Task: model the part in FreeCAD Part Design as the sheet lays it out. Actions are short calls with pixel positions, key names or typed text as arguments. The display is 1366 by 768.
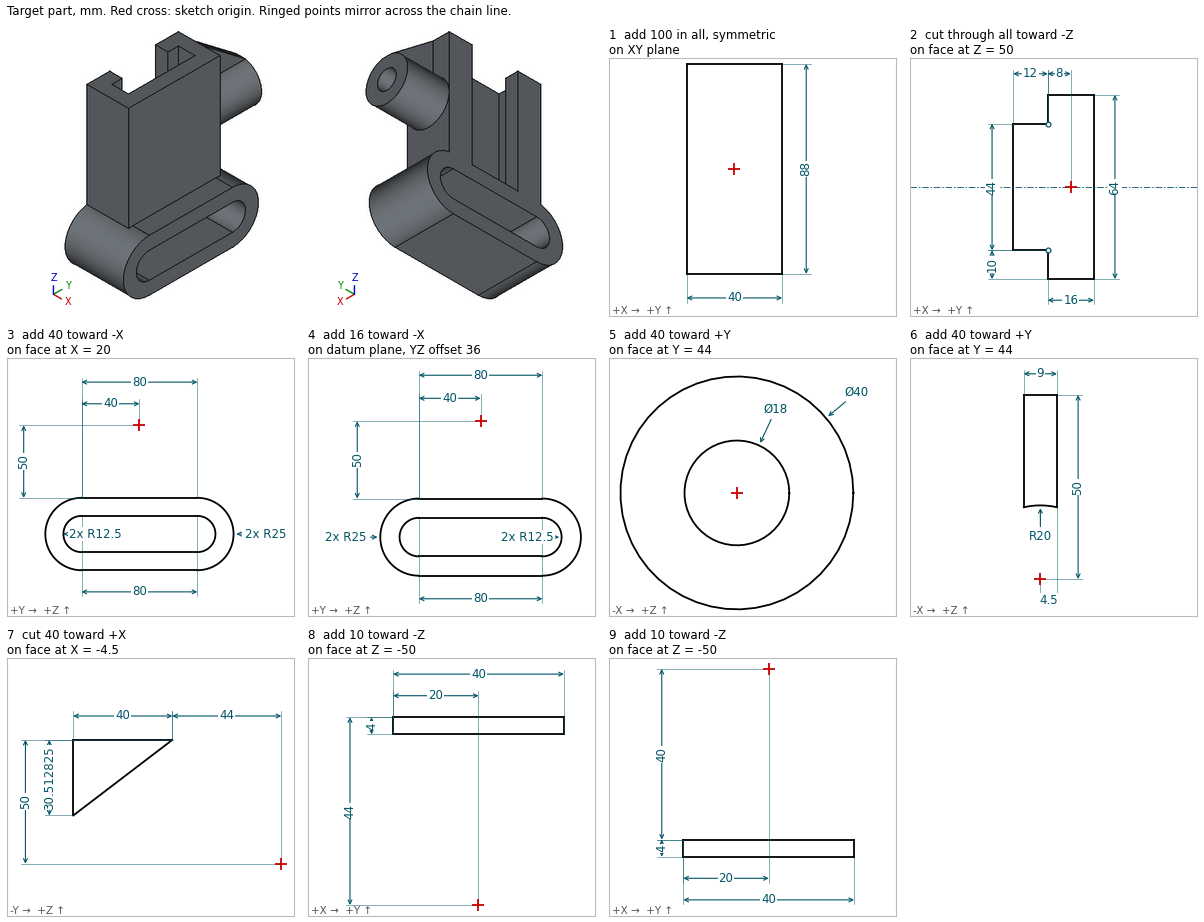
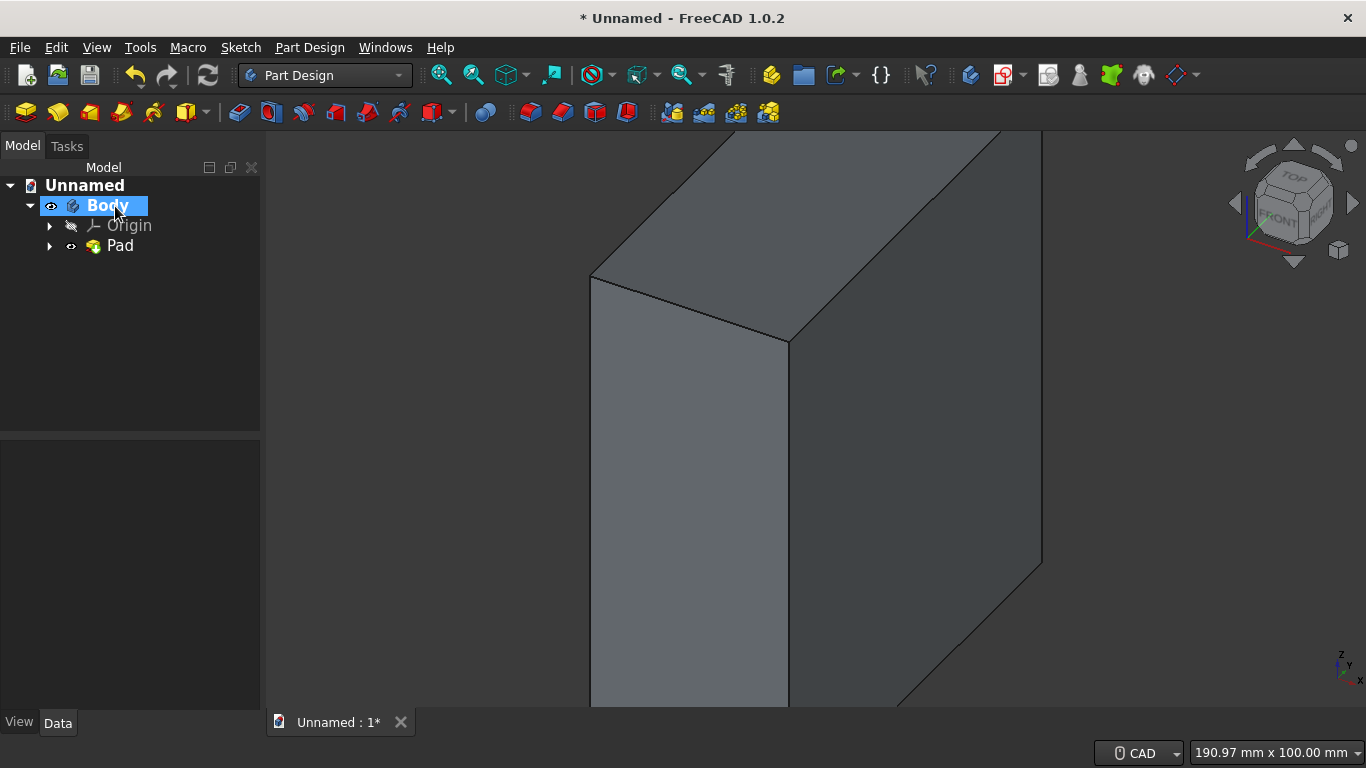
click(442, 76)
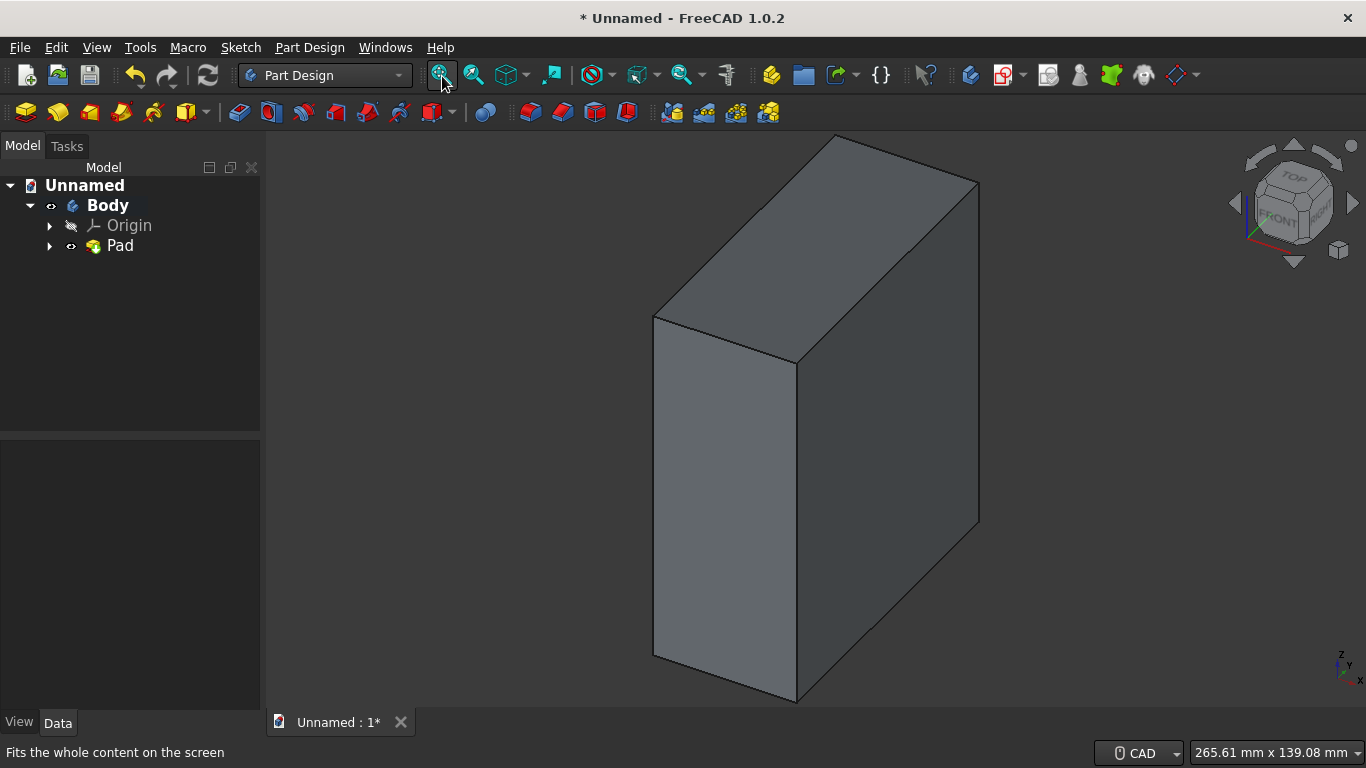
click(842, 223)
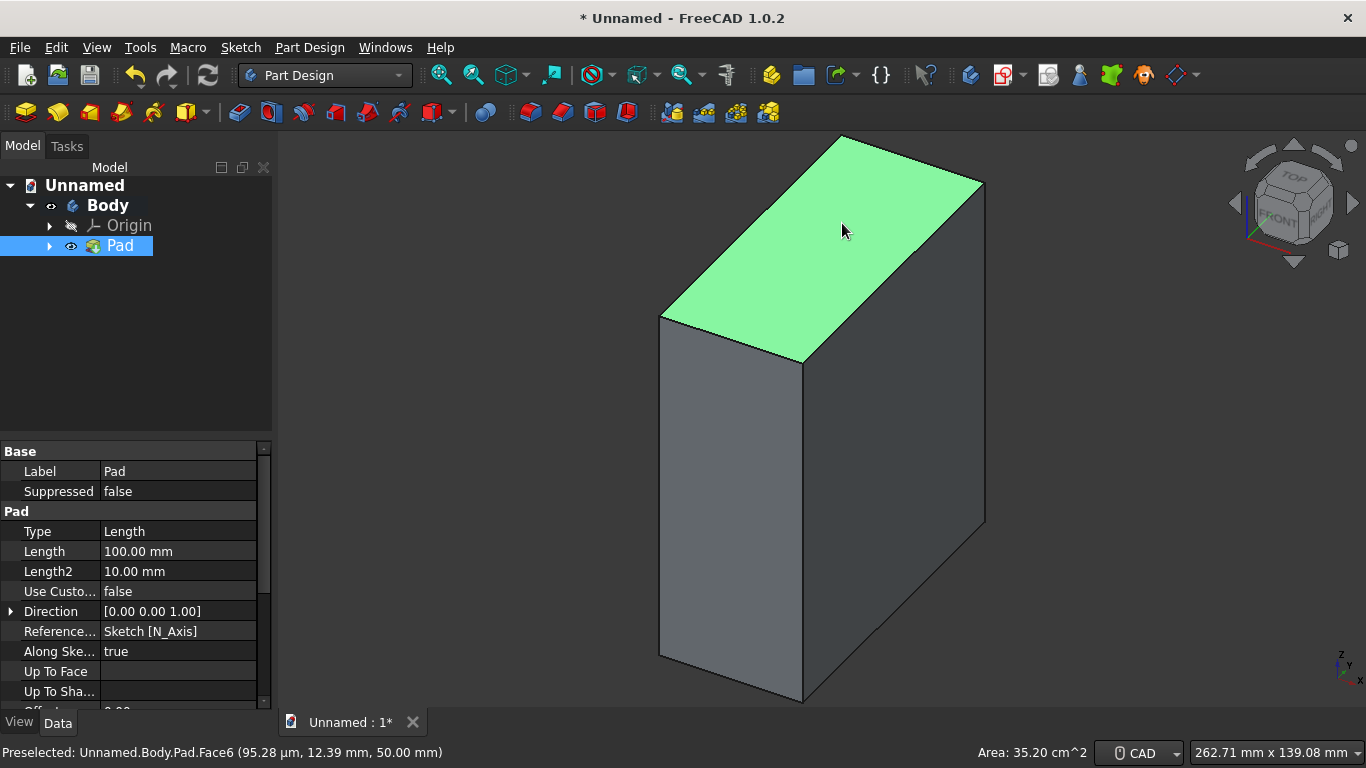
click(1004, 76)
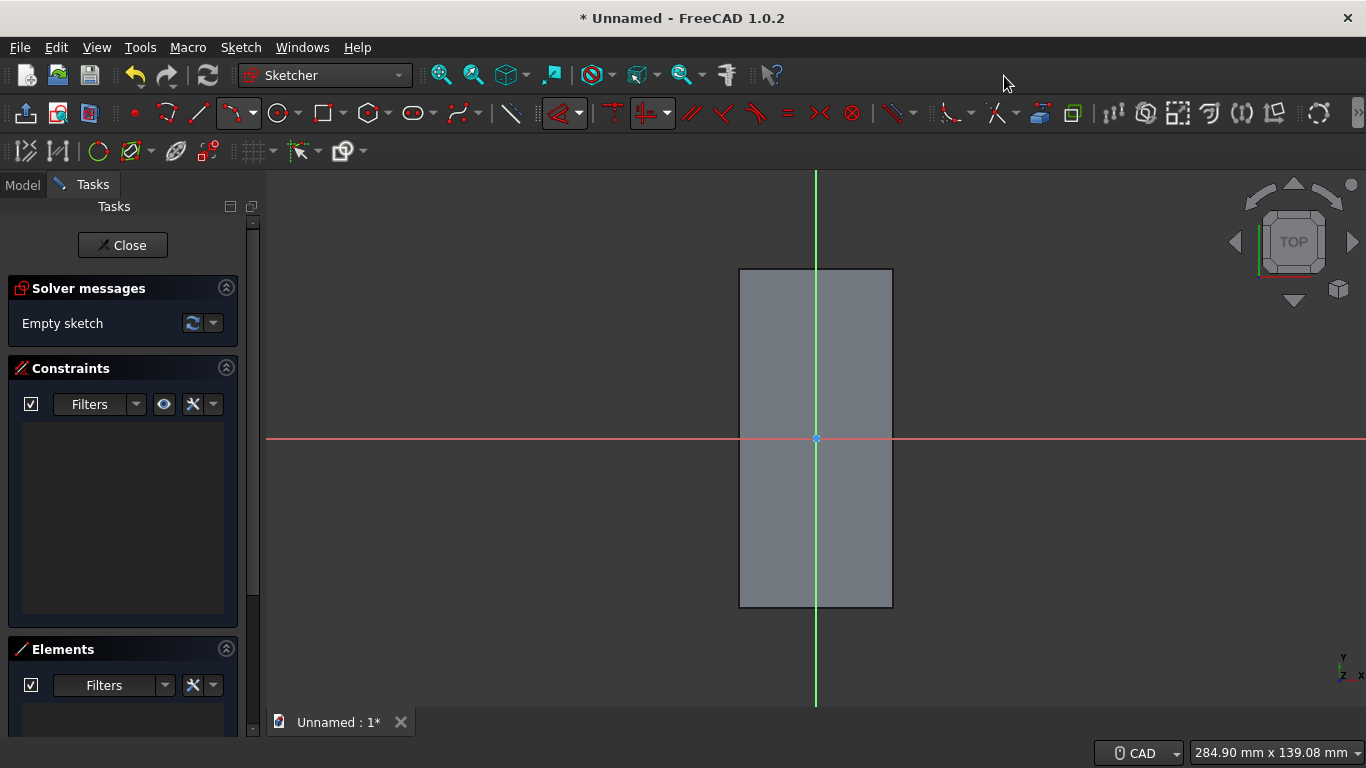
scroll(885, 439, up, 2)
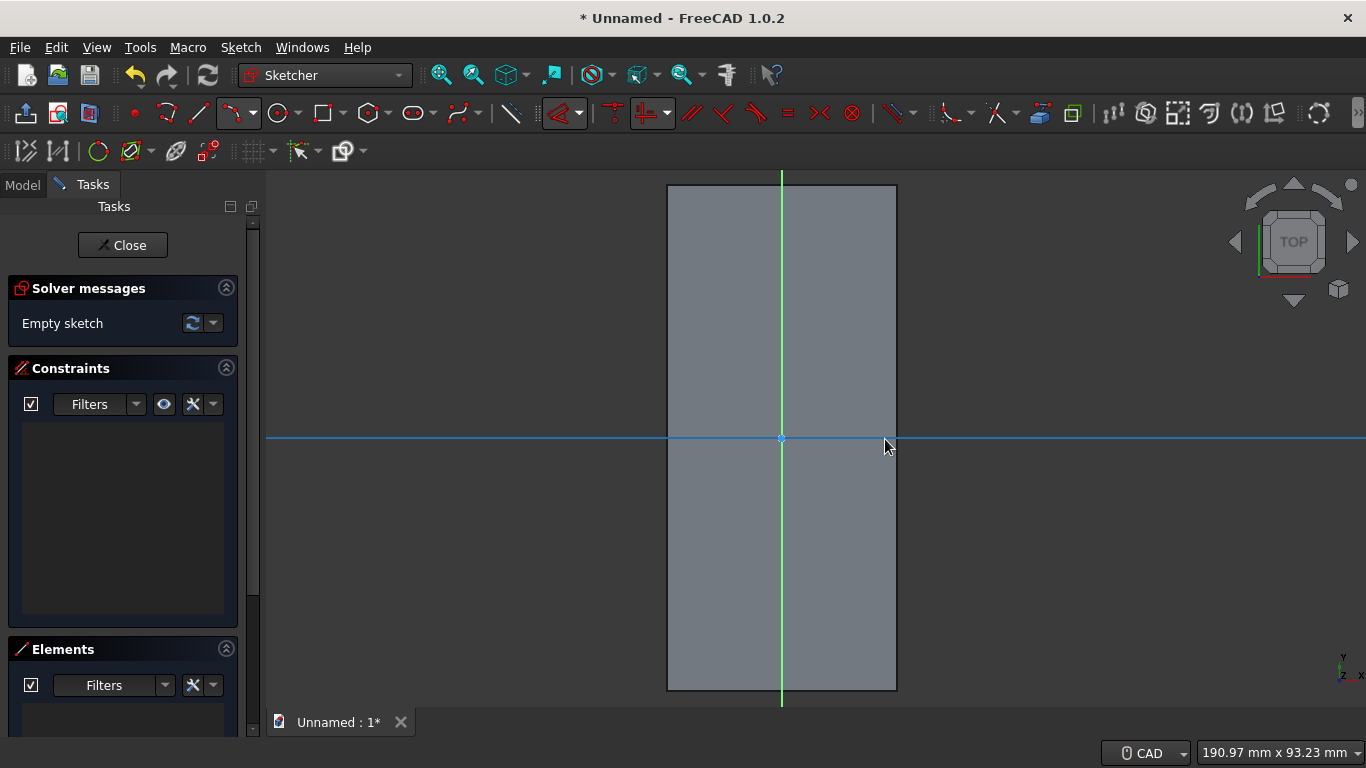
key(g)
key(m)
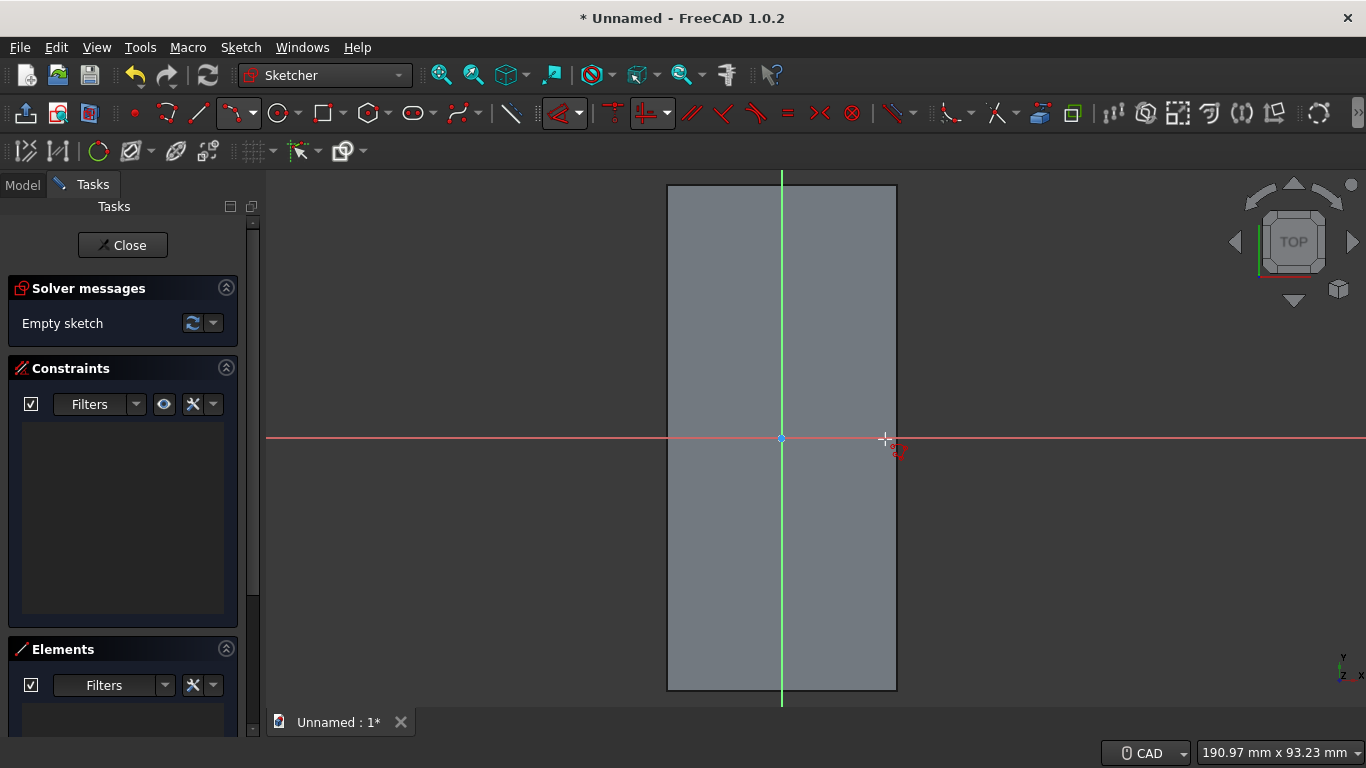
click(736, 311)
click(667, 311)
click(667, 565)
click(736, 565)
click(736, 622)
click(828, 622)
click(828, 254)
click(736, 254)
click(736, 312)
key(Escape)
key(Escape)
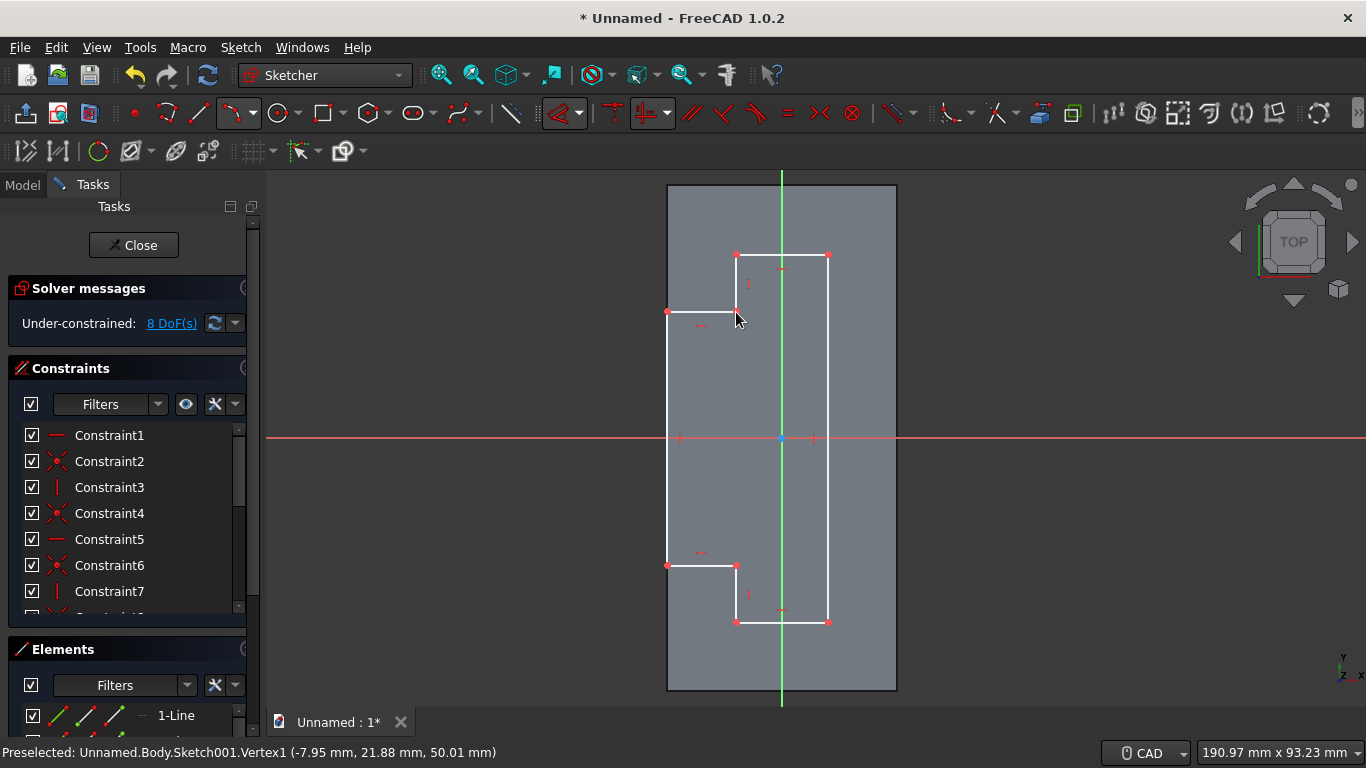
click(736, 312)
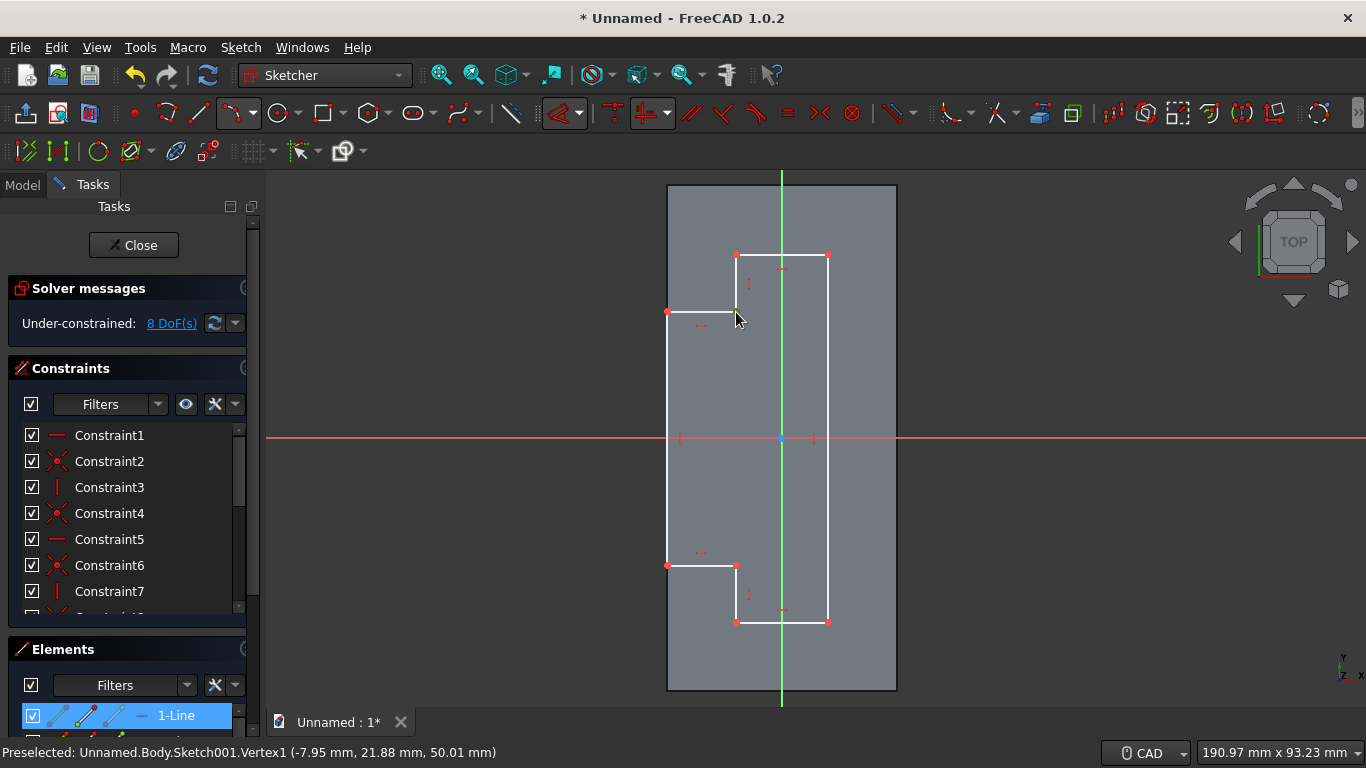
click(736, 566)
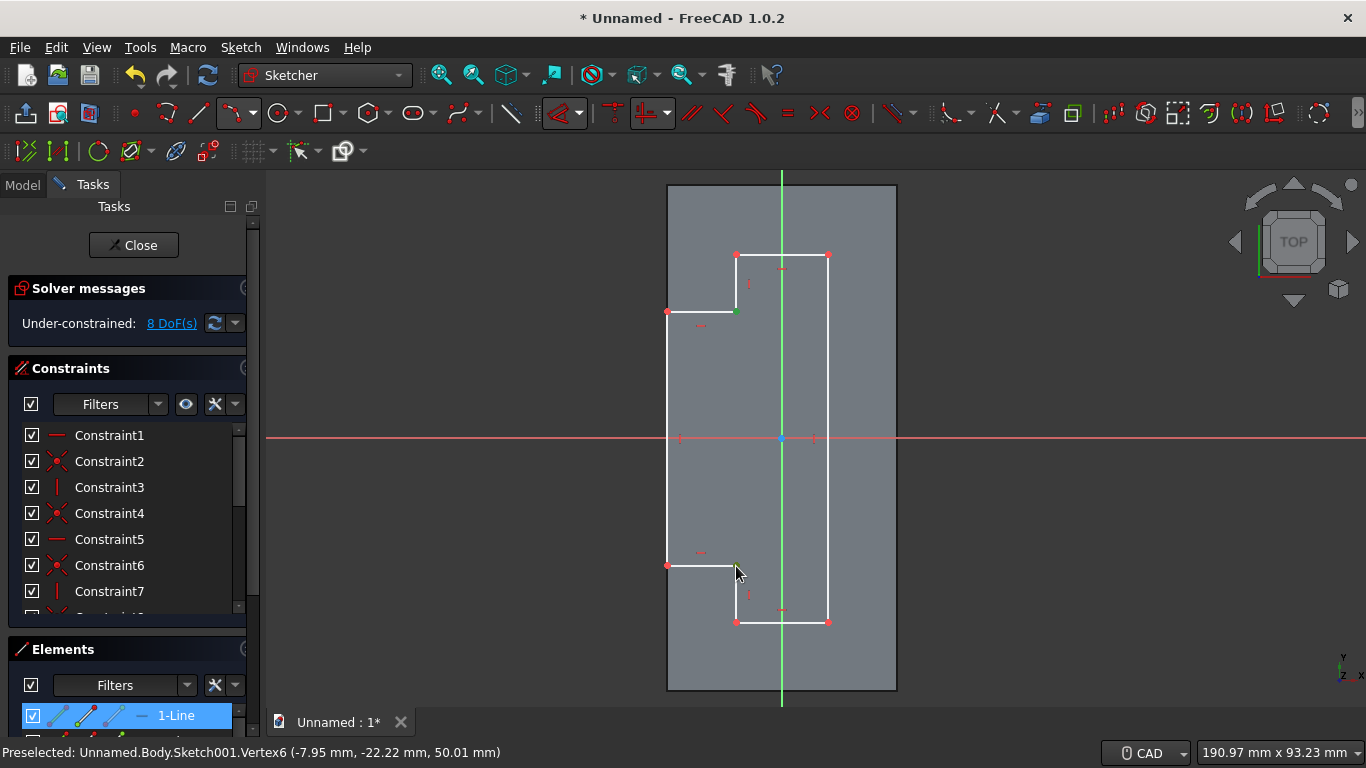
click(359, 438)